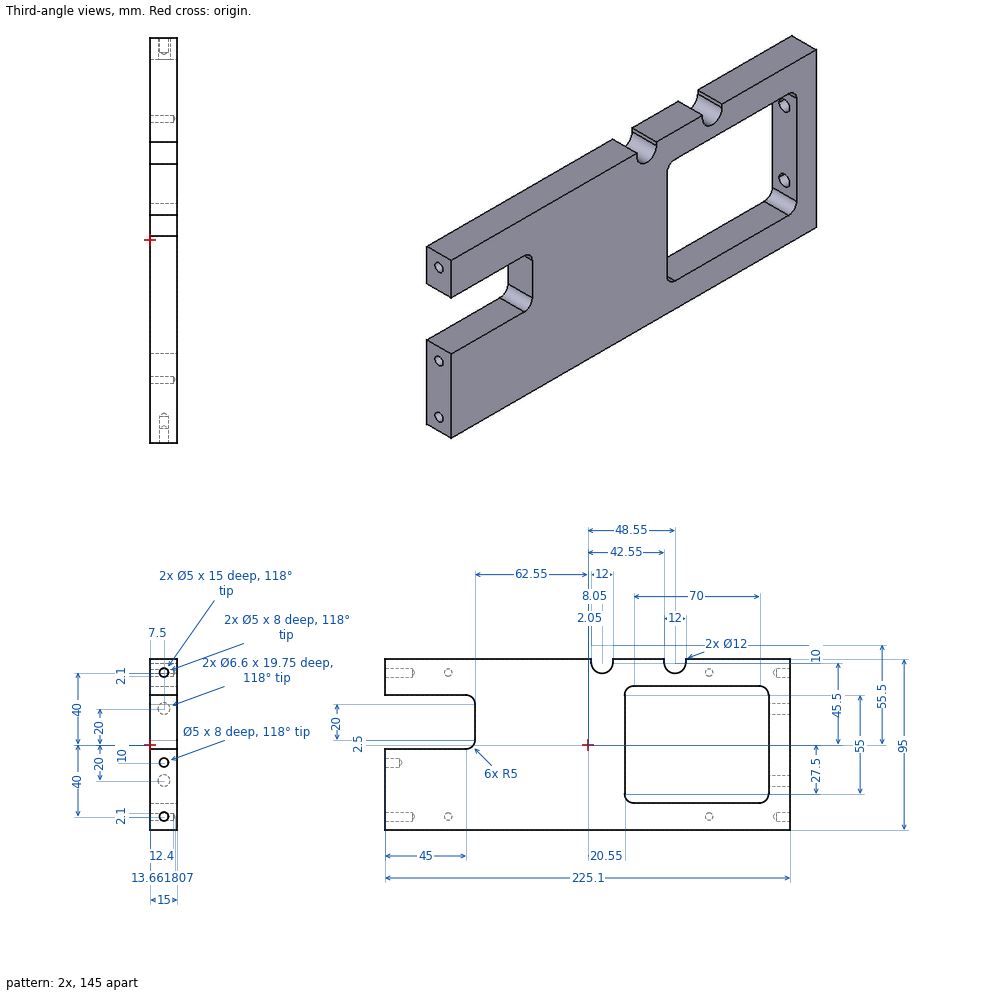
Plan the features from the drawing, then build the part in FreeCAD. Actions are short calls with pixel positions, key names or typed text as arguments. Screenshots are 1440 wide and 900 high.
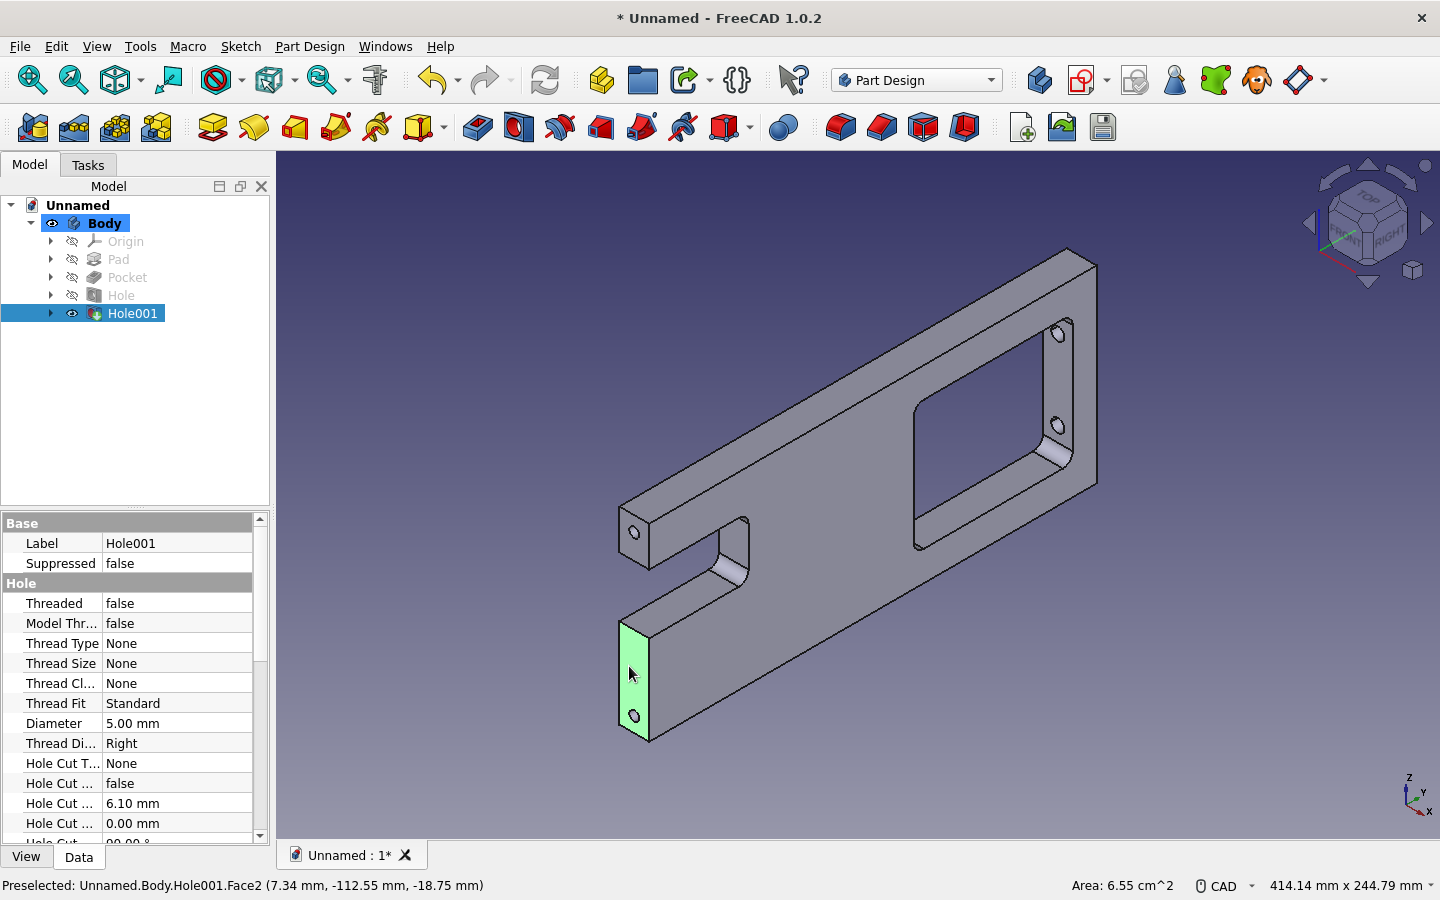
click(1080, 80)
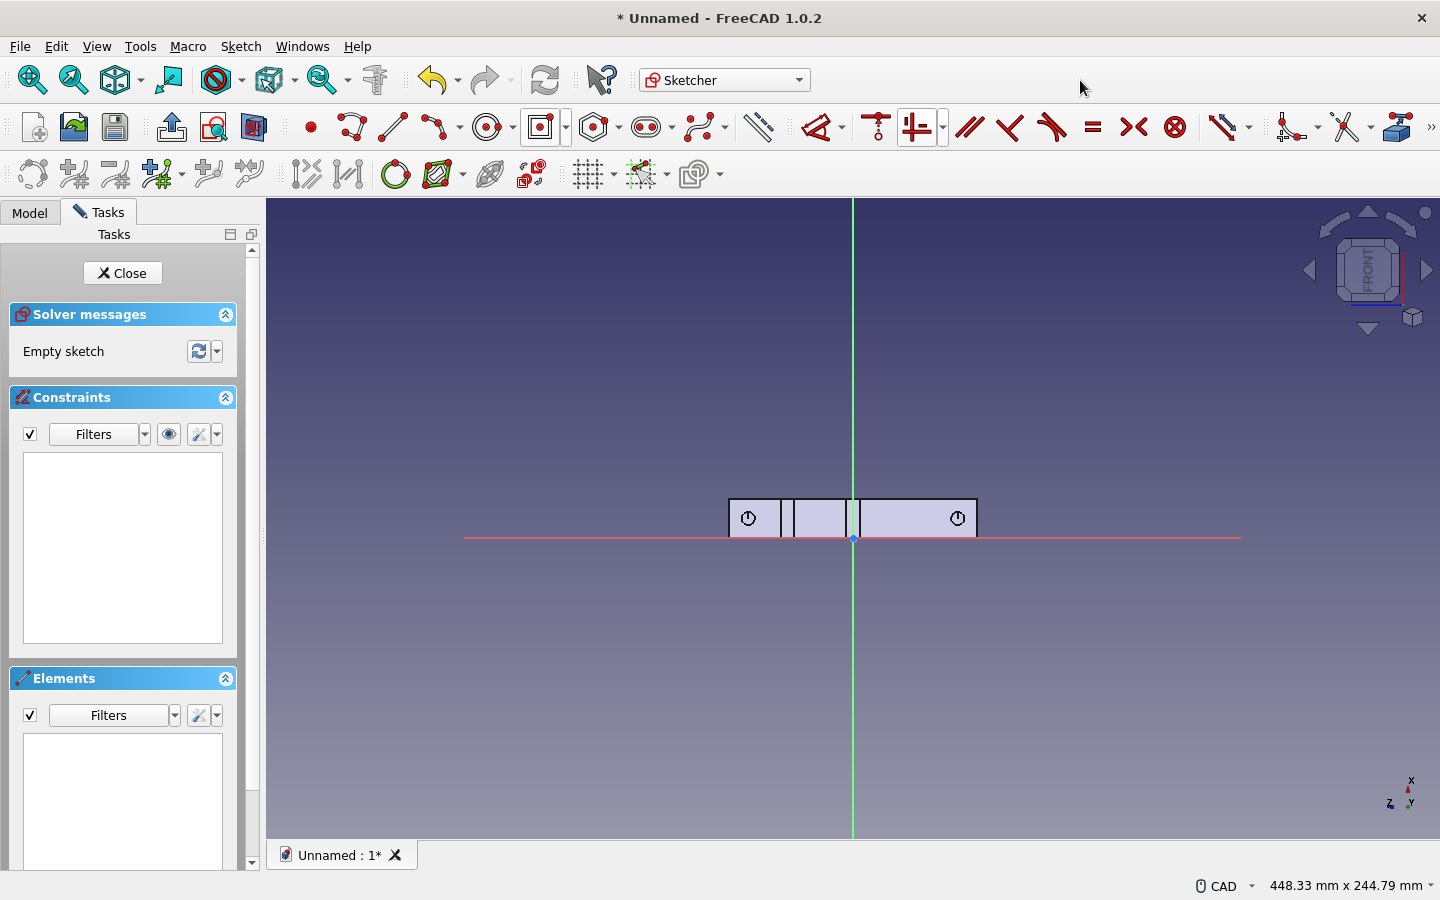
scroll(884, 519, up, 15)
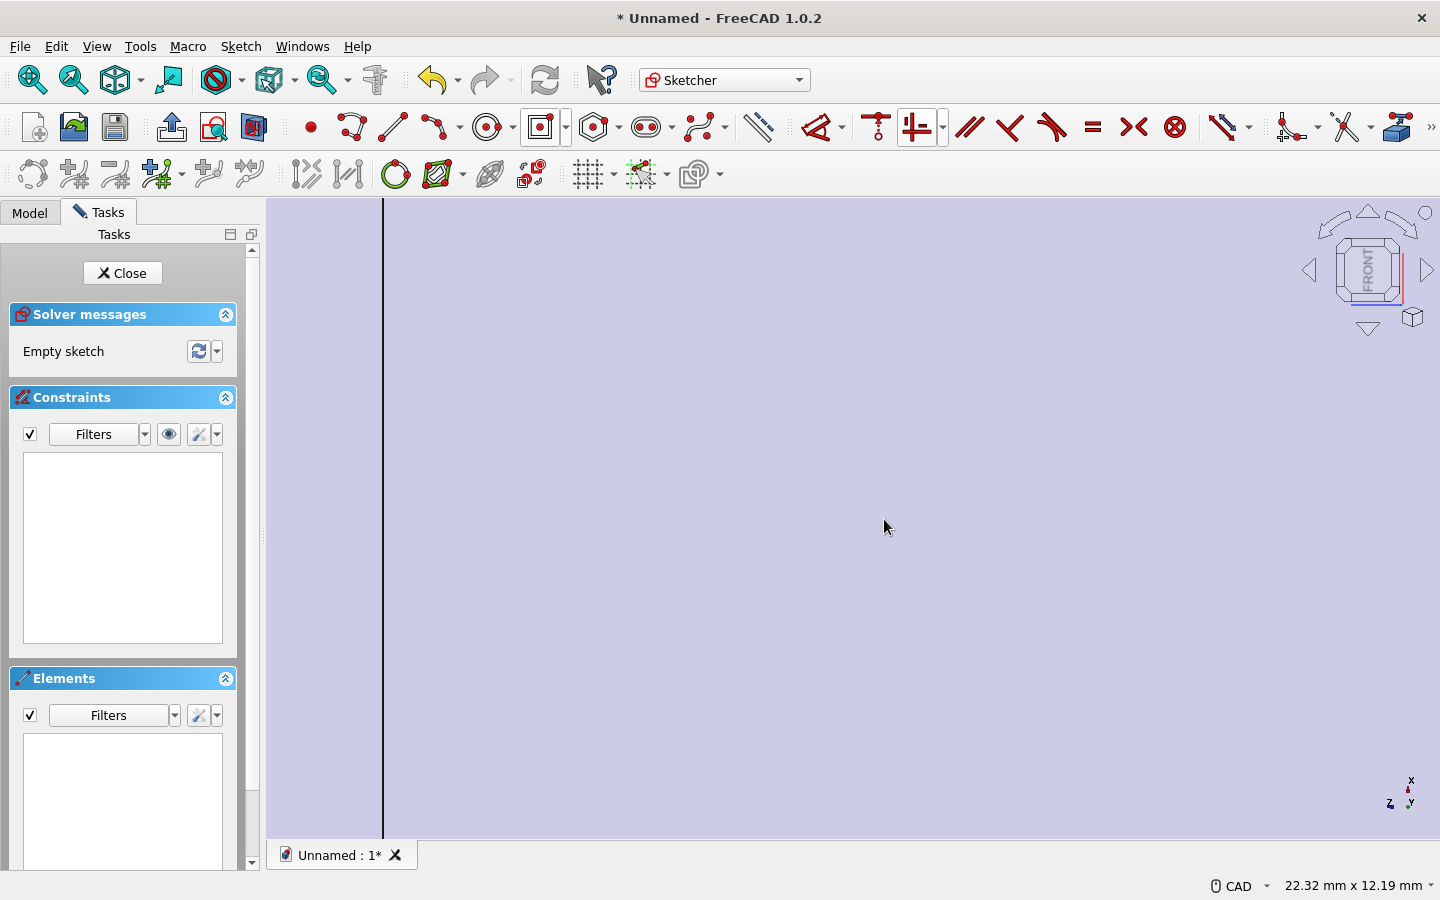
scroll(763, 461, up, 2)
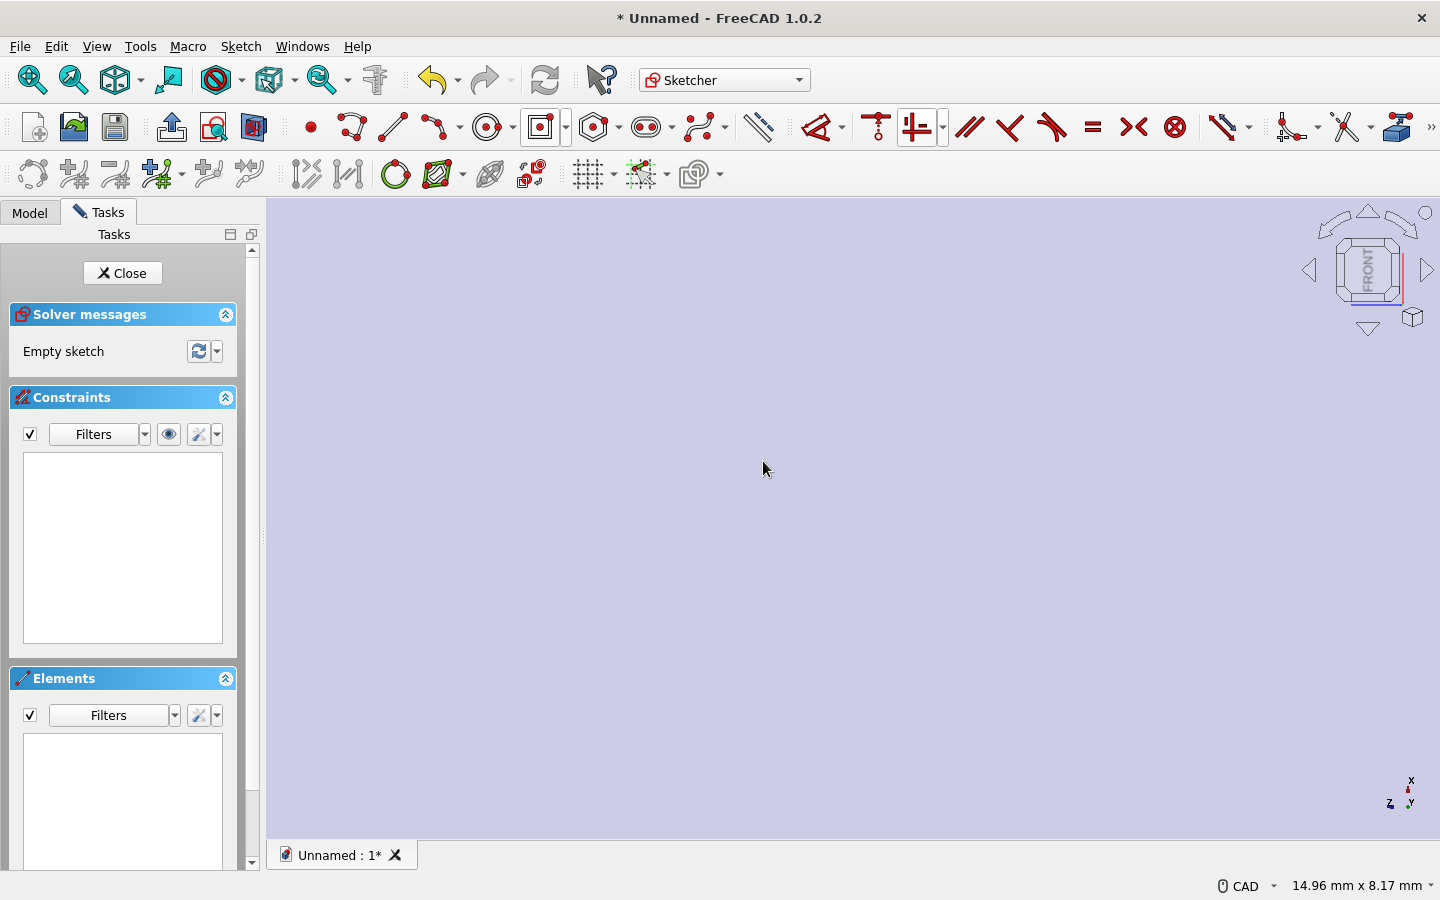
click(486, 128)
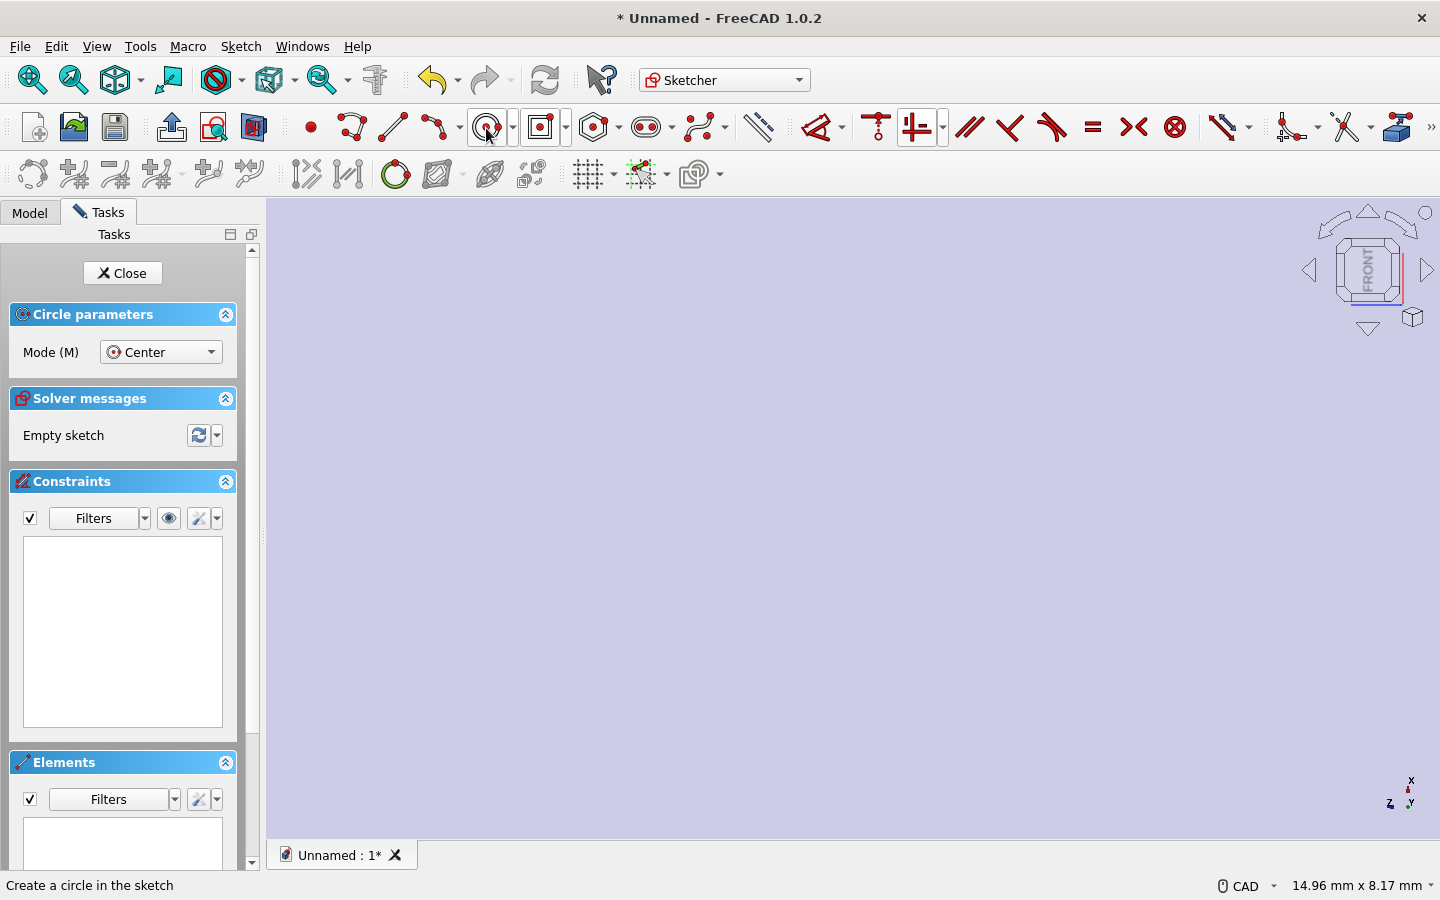
click(784, 518)
move(923, 379)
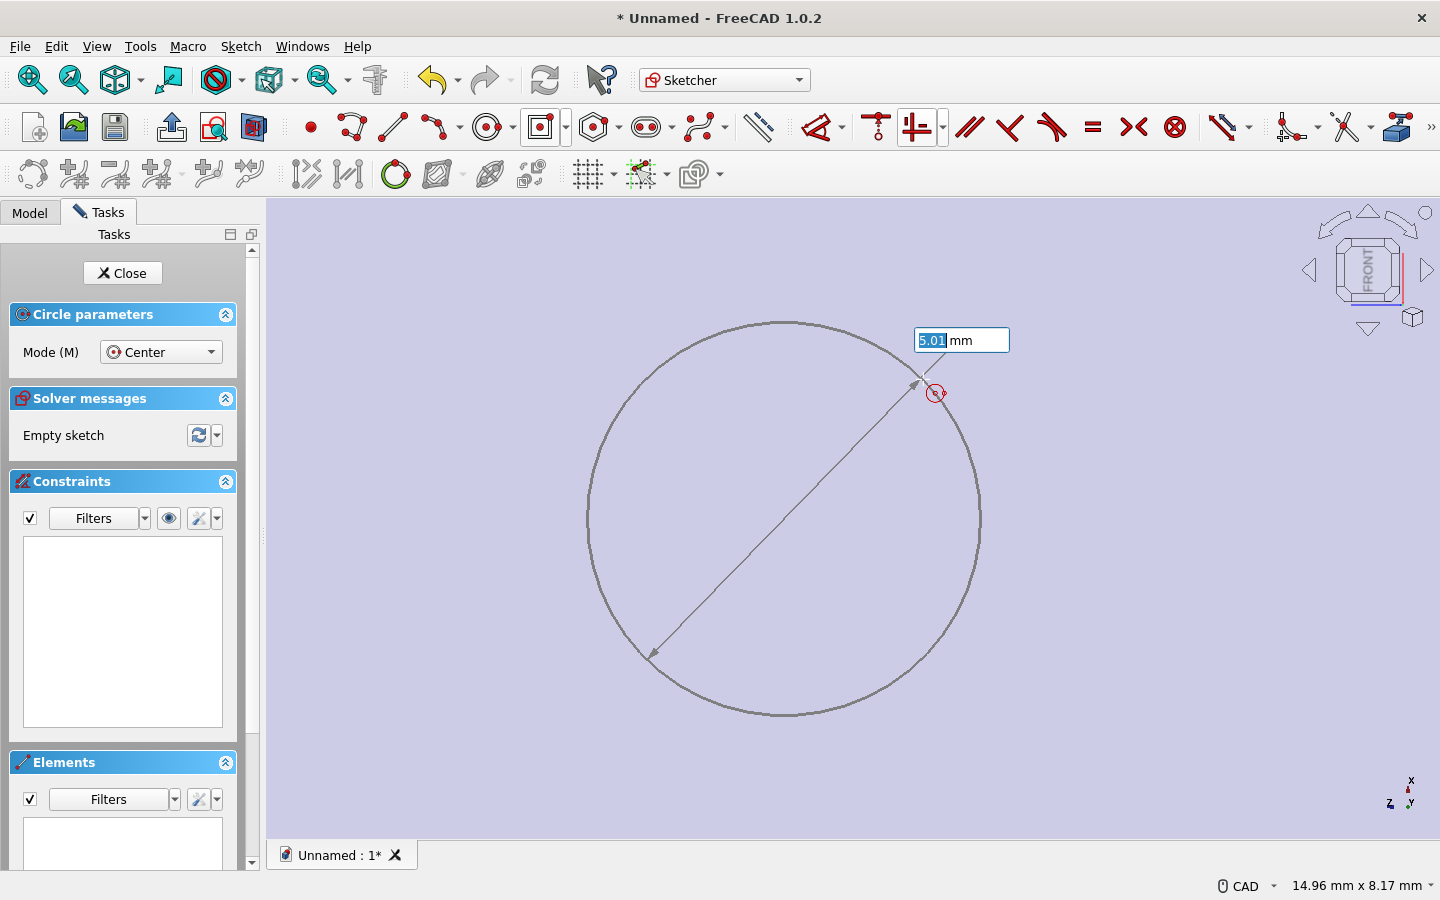
text(5)
key(Return)
key(Escape)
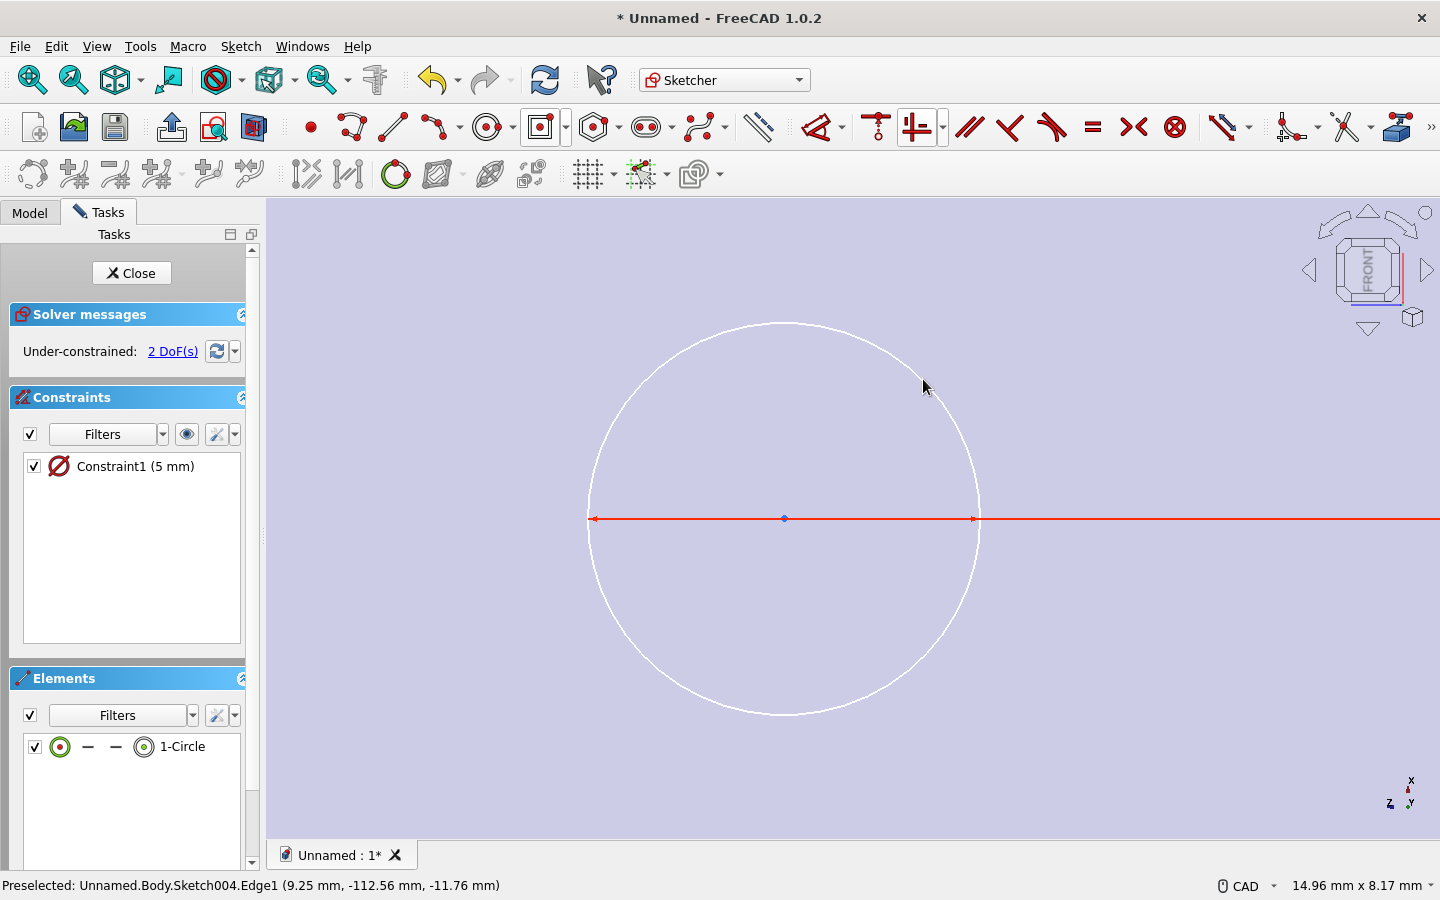
click(816, 128)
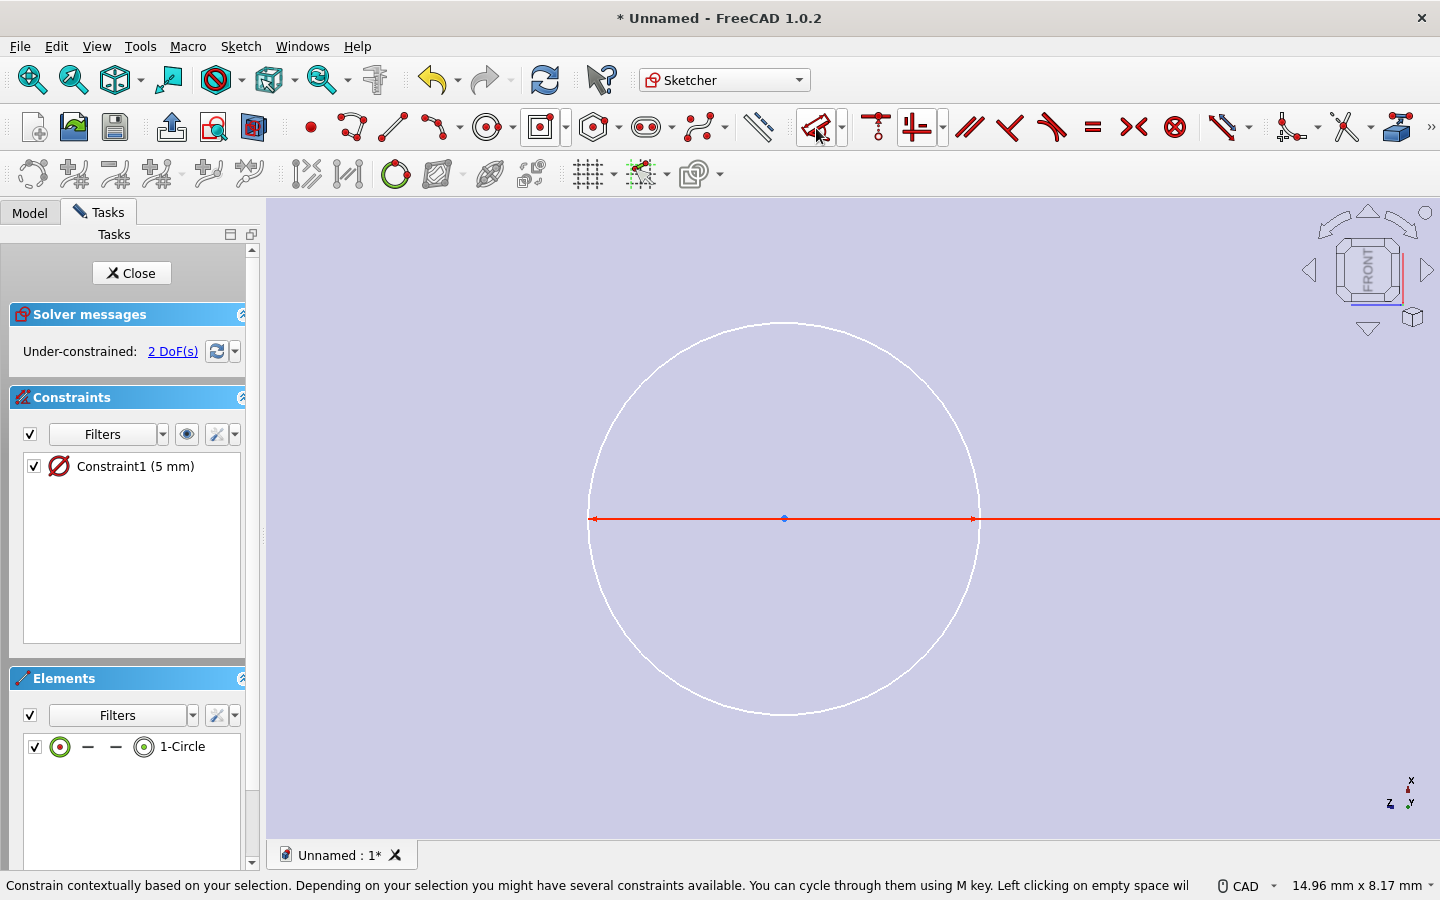
click(784, 519)
click(539, 485)